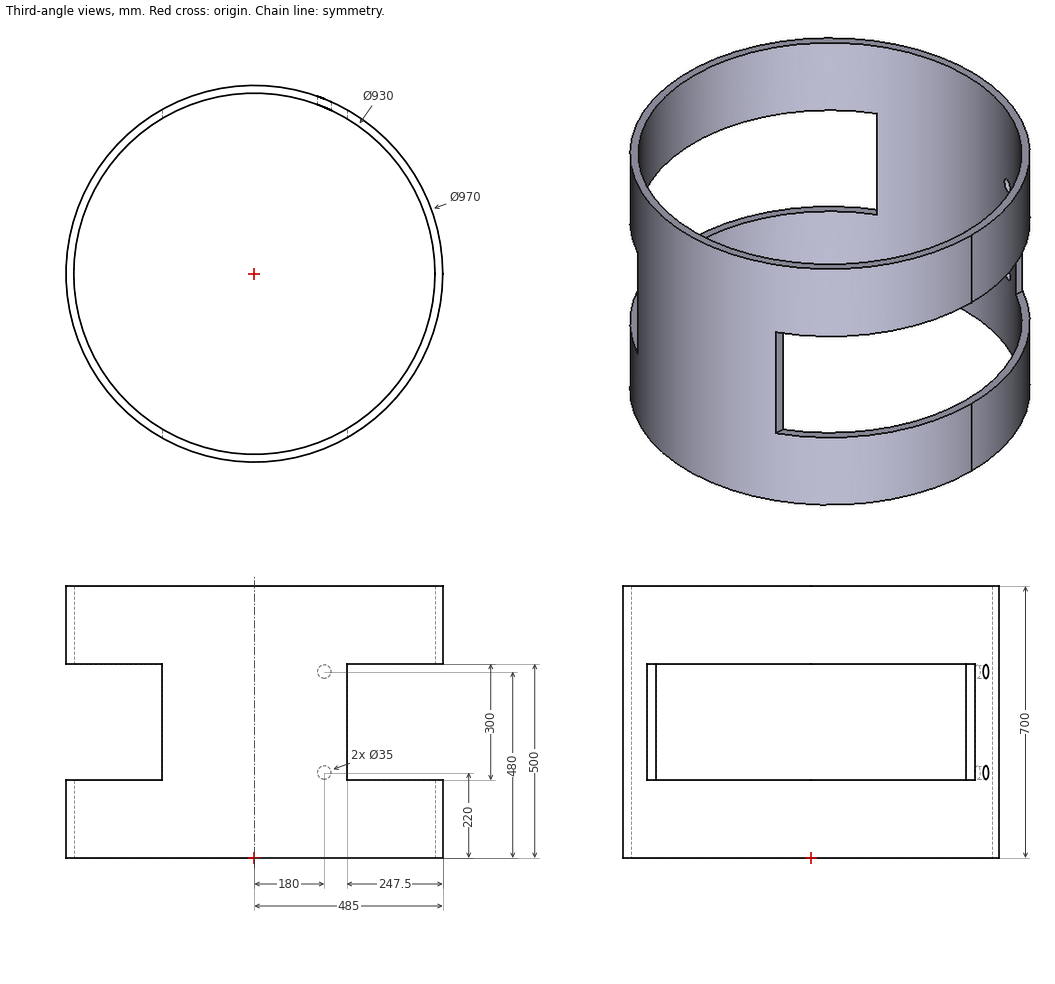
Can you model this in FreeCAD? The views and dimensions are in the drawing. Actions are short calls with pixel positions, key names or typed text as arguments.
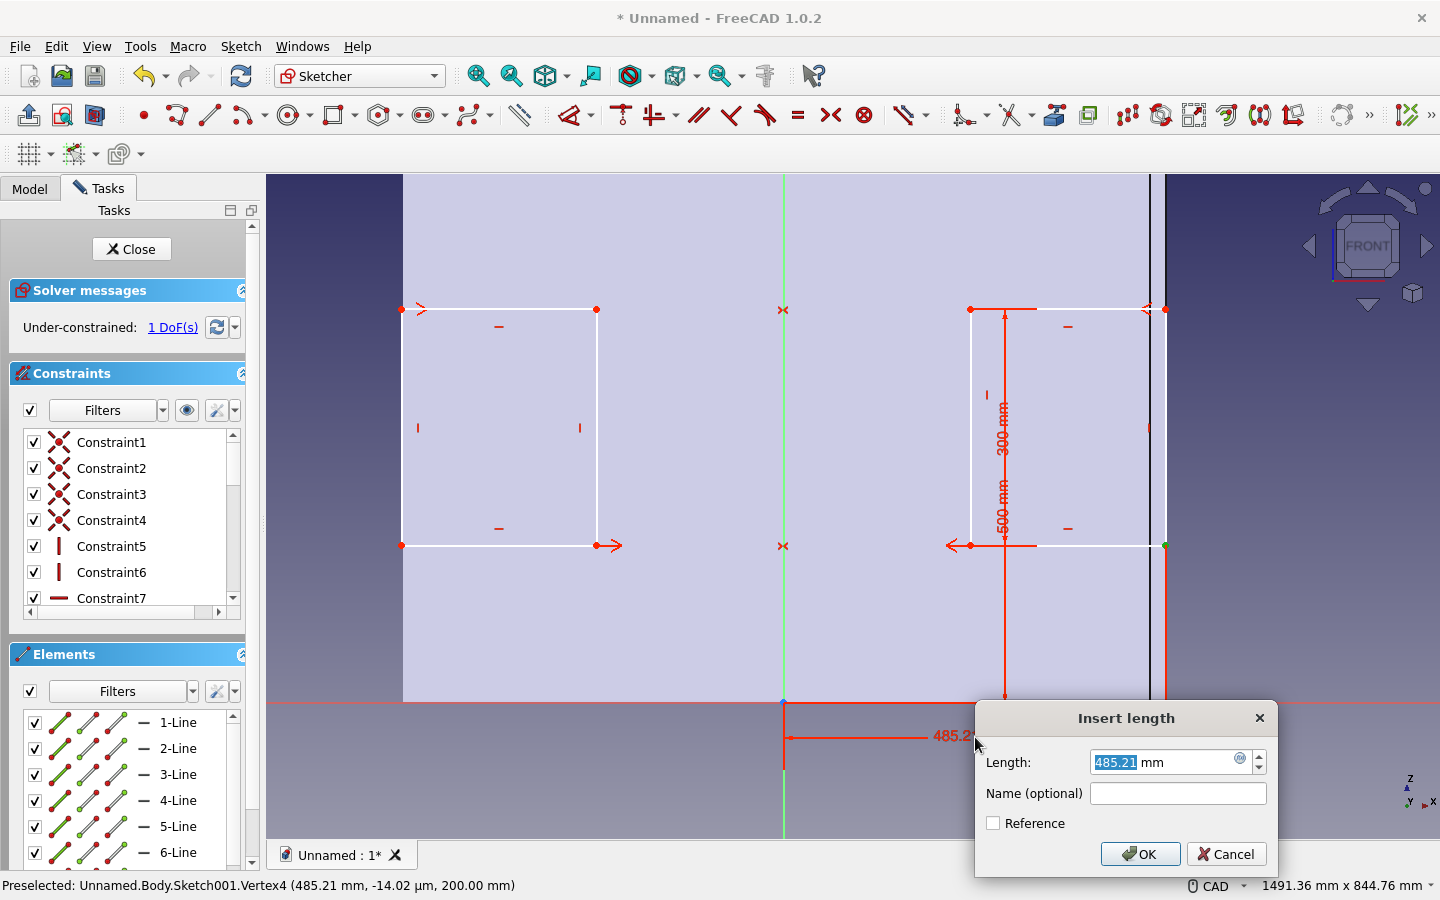
text(485)
key(Return)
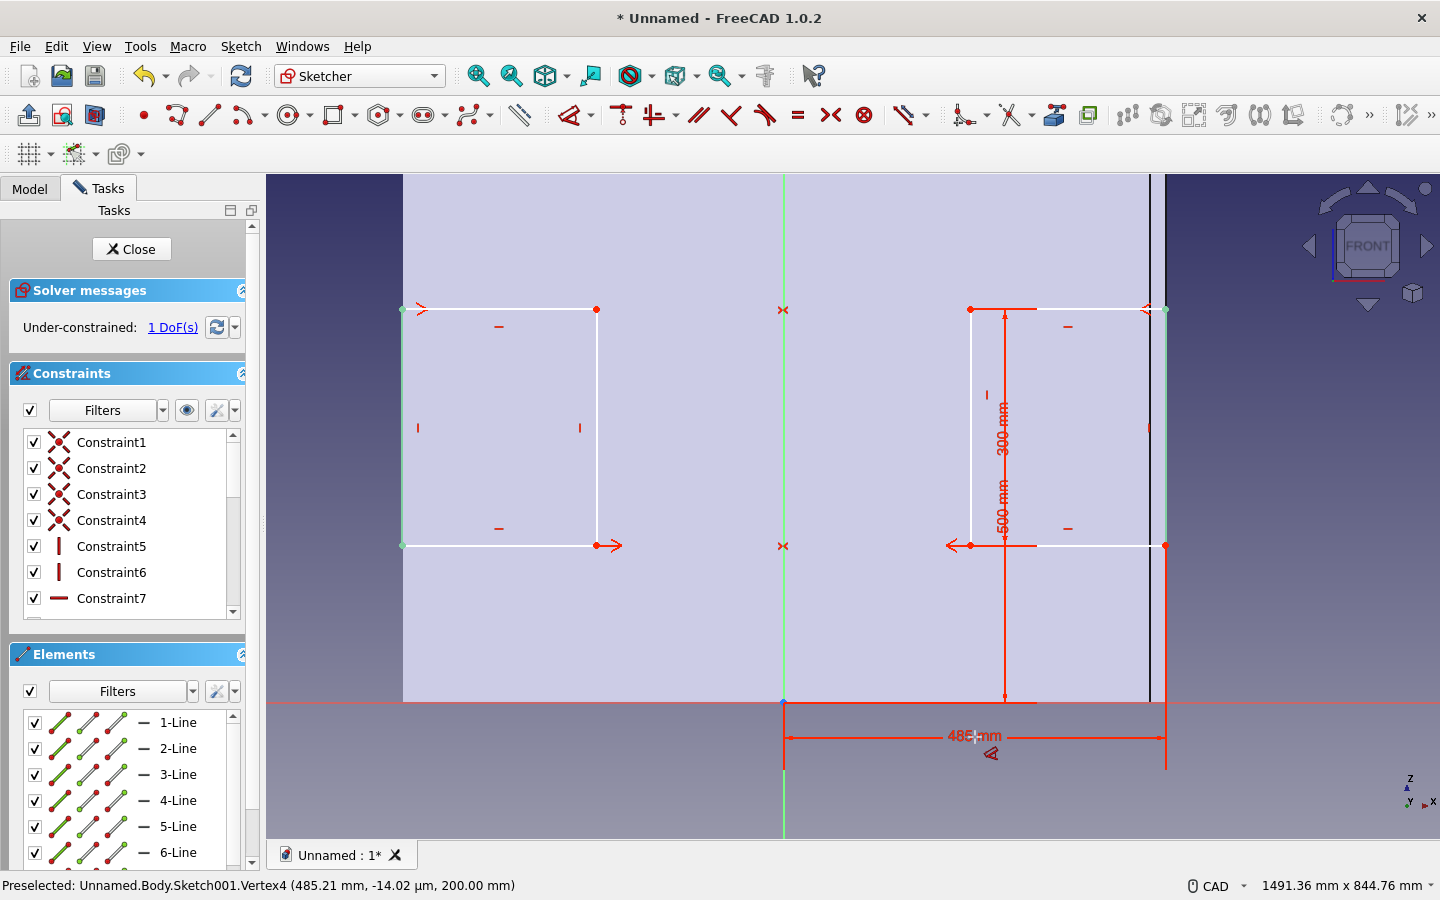
click(1029, 546)
click(1068, 580)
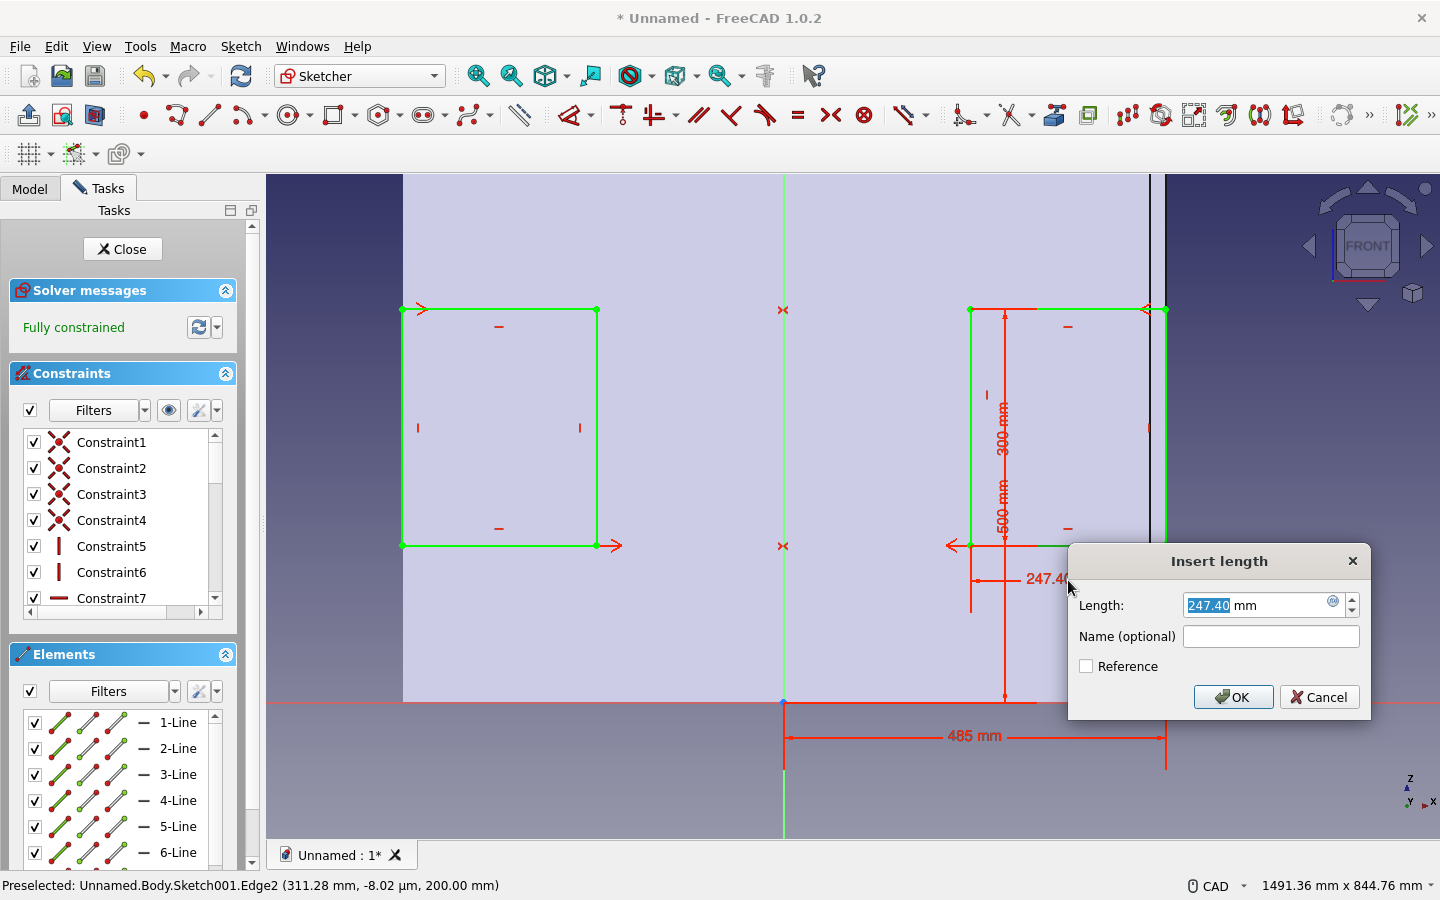
text(247.5)
key(Return)
key(Escape)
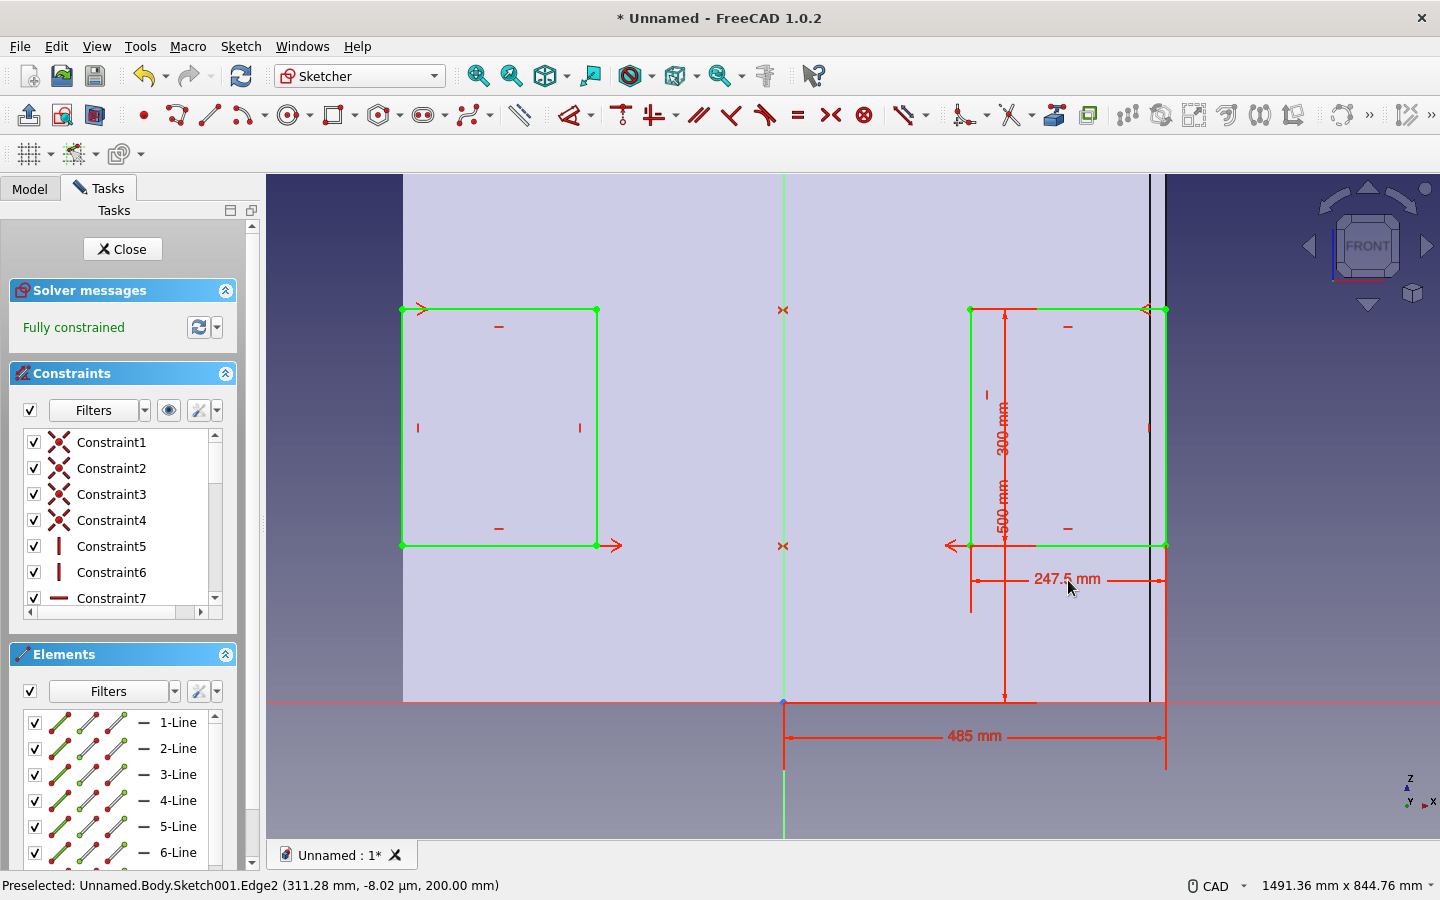
click(123, 249)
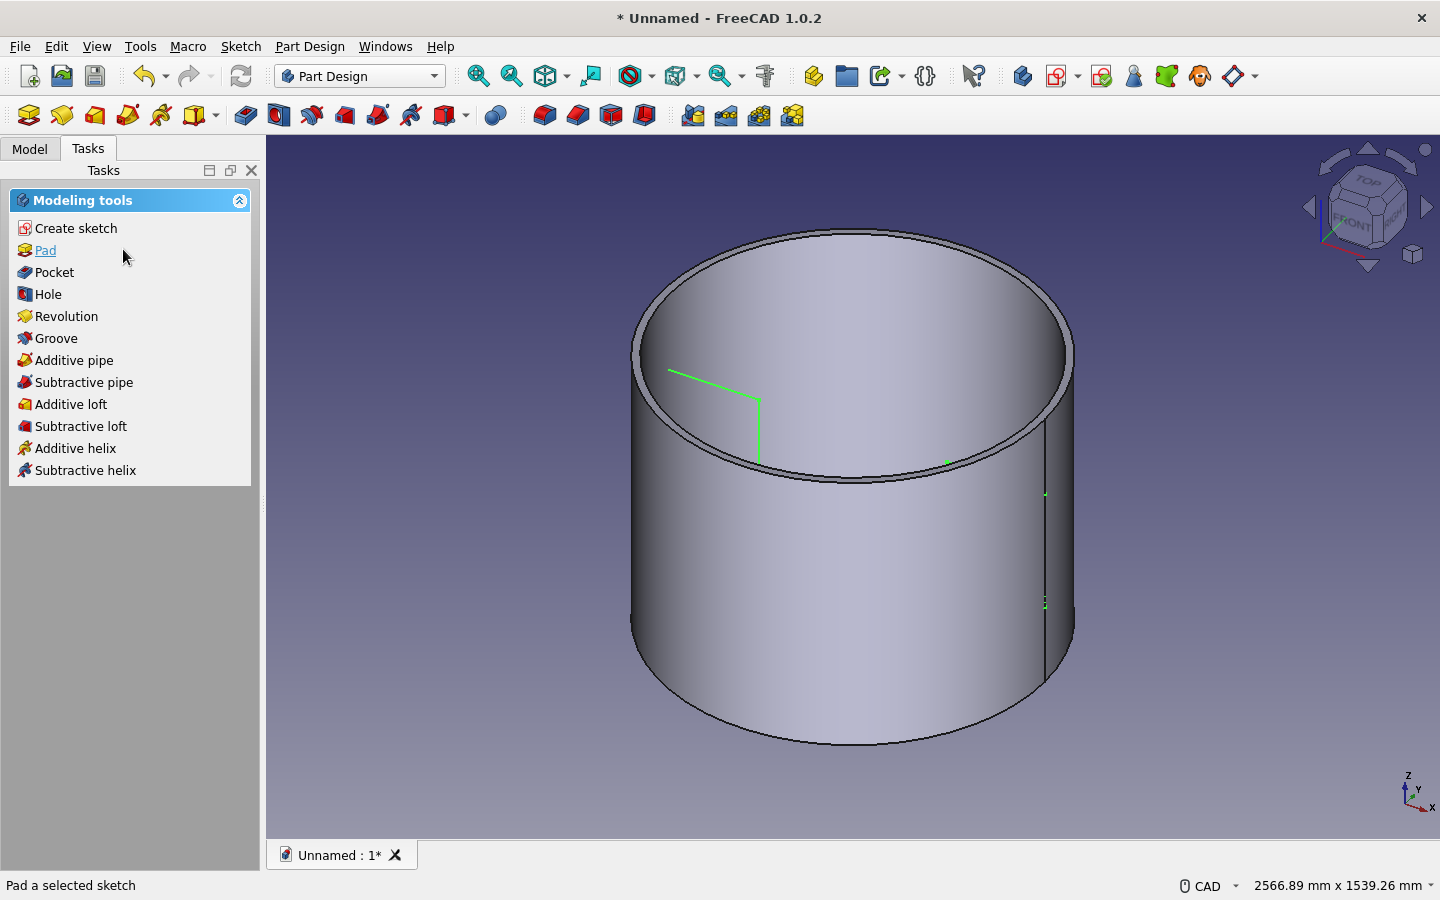
click(246, 116)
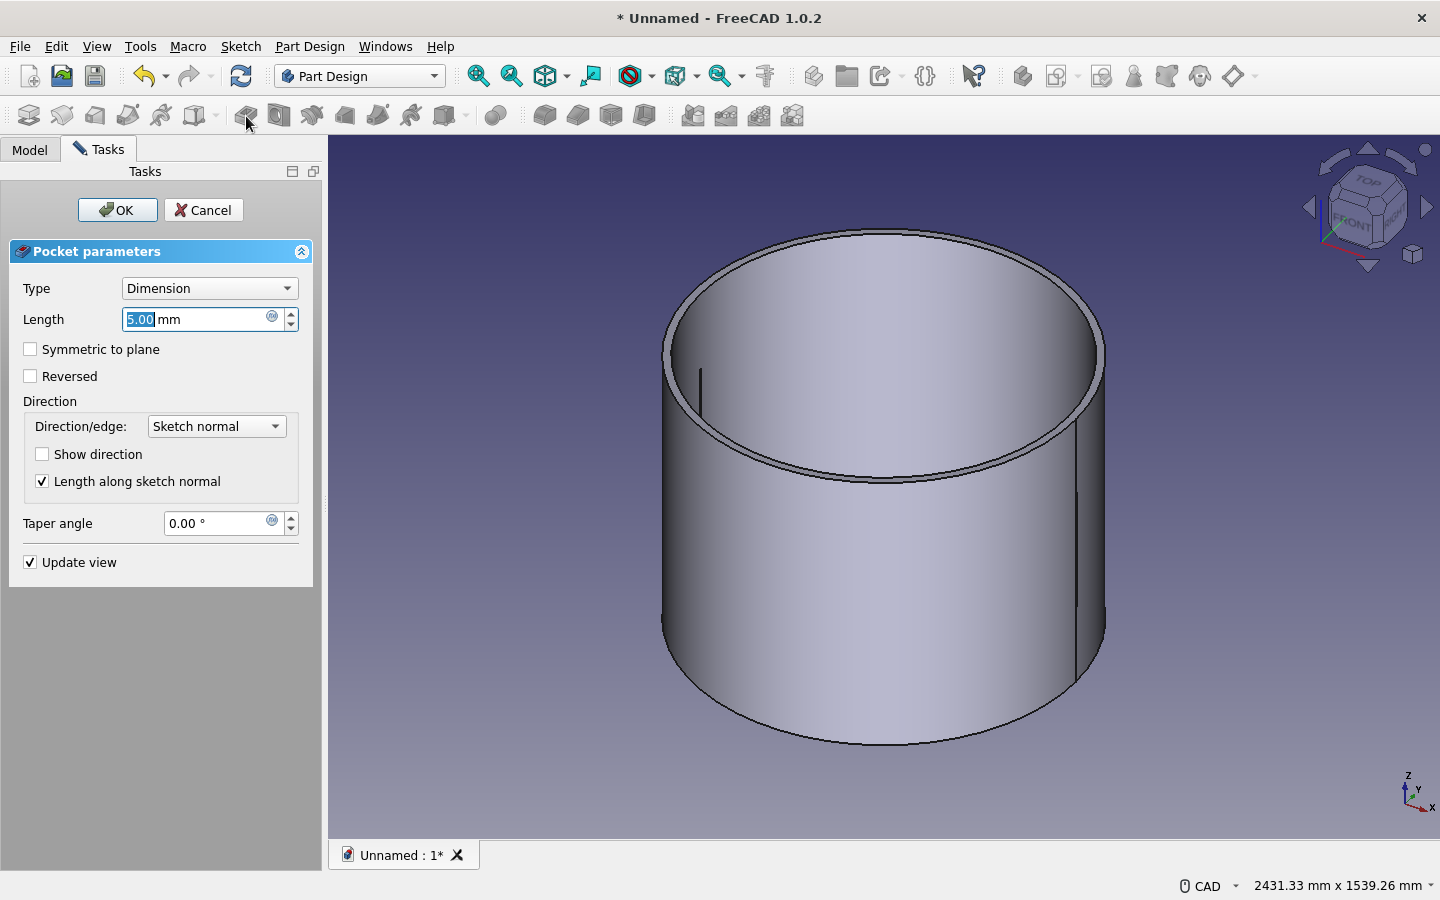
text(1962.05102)
key(Tab)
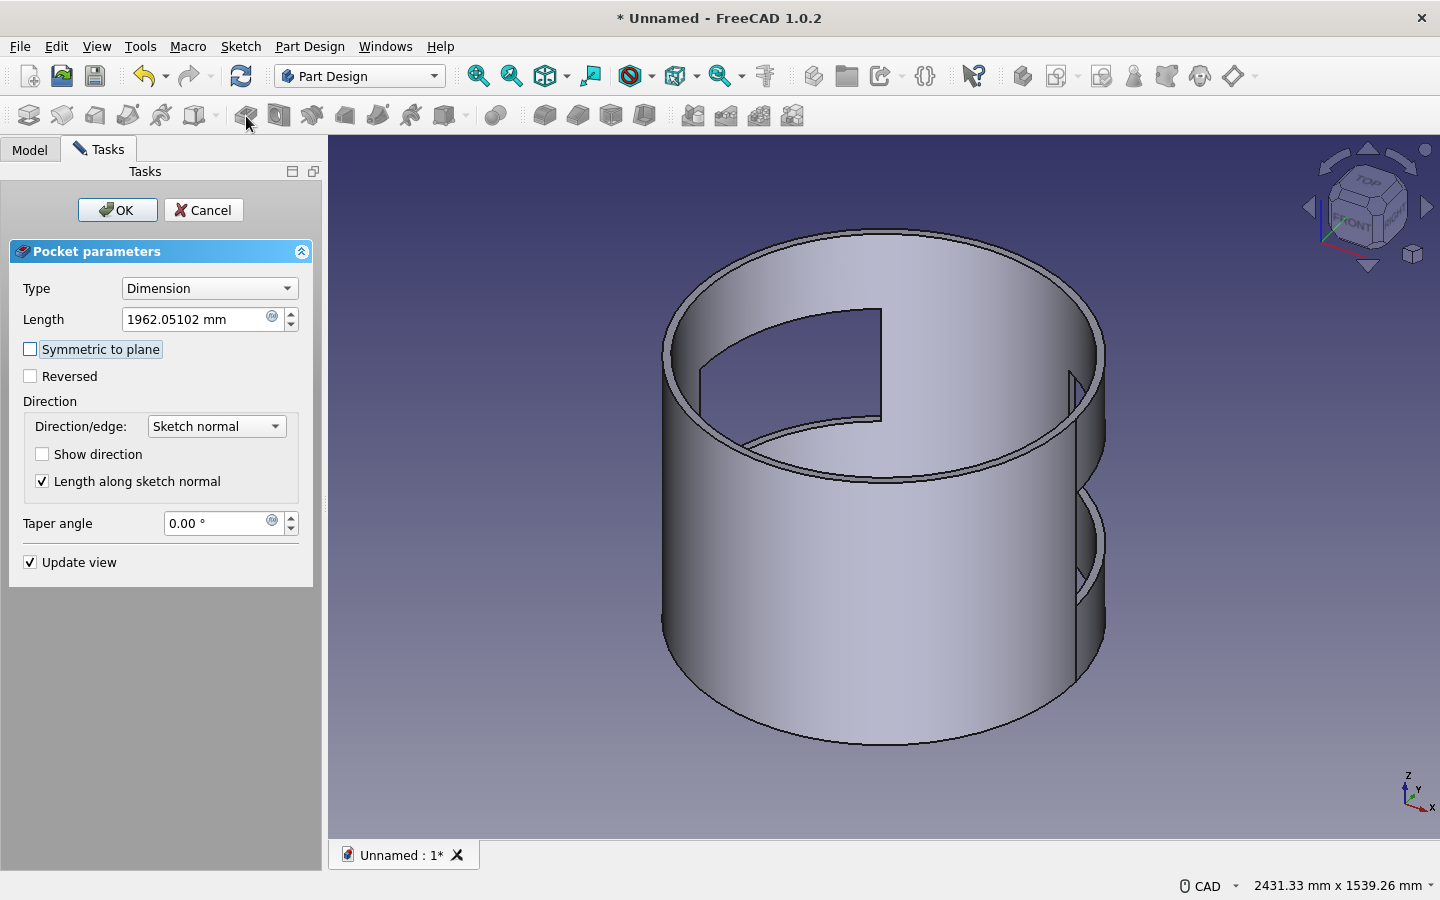
click(31, 349)